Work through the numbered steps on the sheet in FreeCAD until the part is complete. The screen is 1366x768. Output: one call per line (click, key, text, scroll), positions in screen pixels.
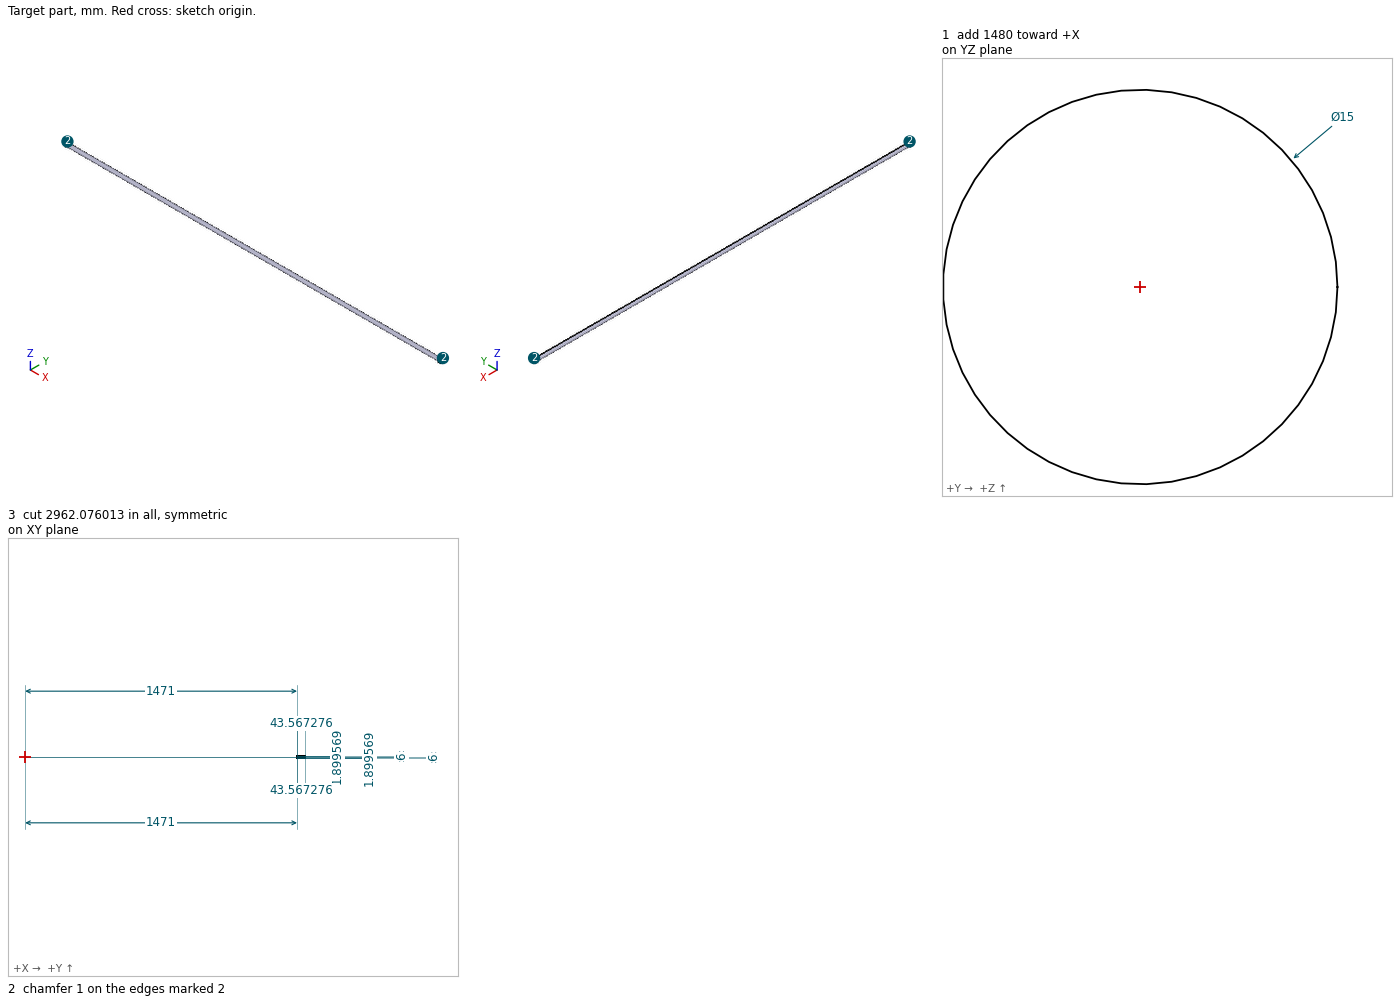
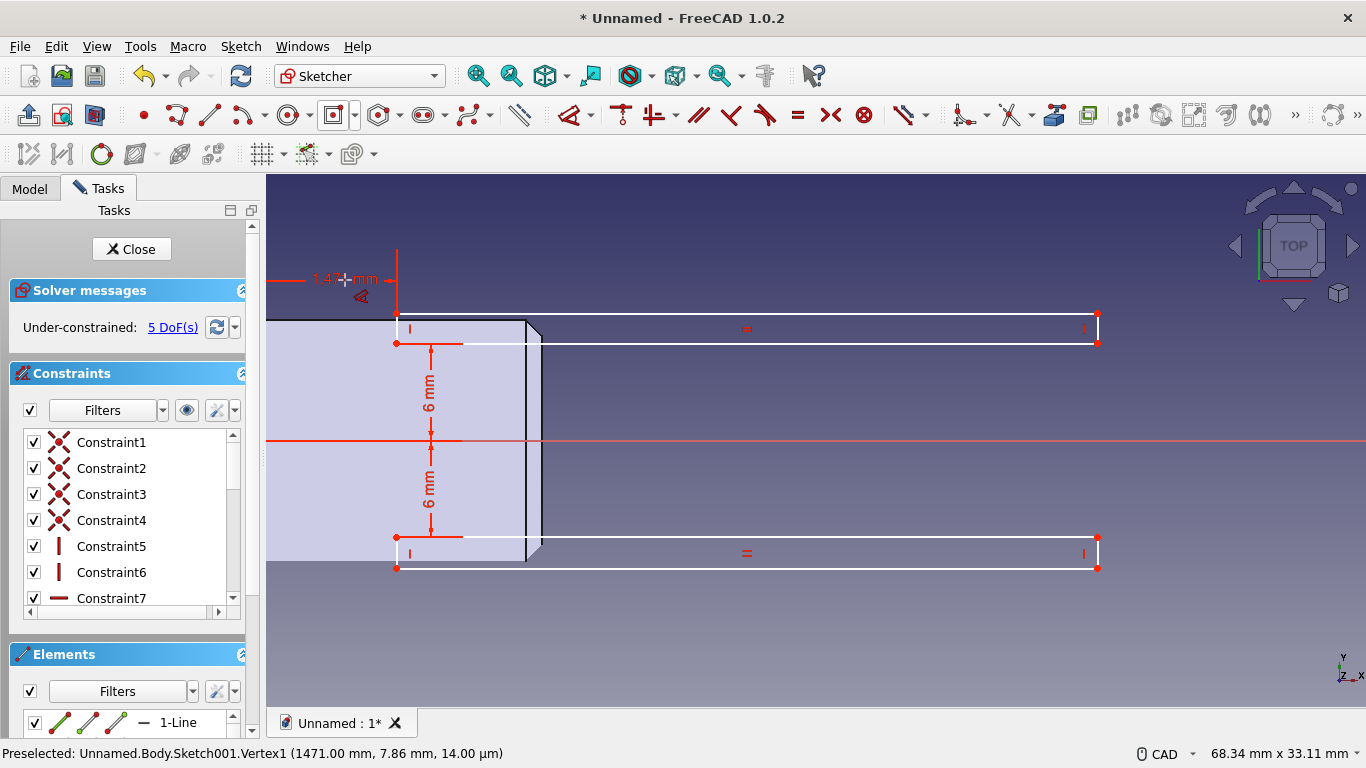
click(397, 537)
click(345, 571)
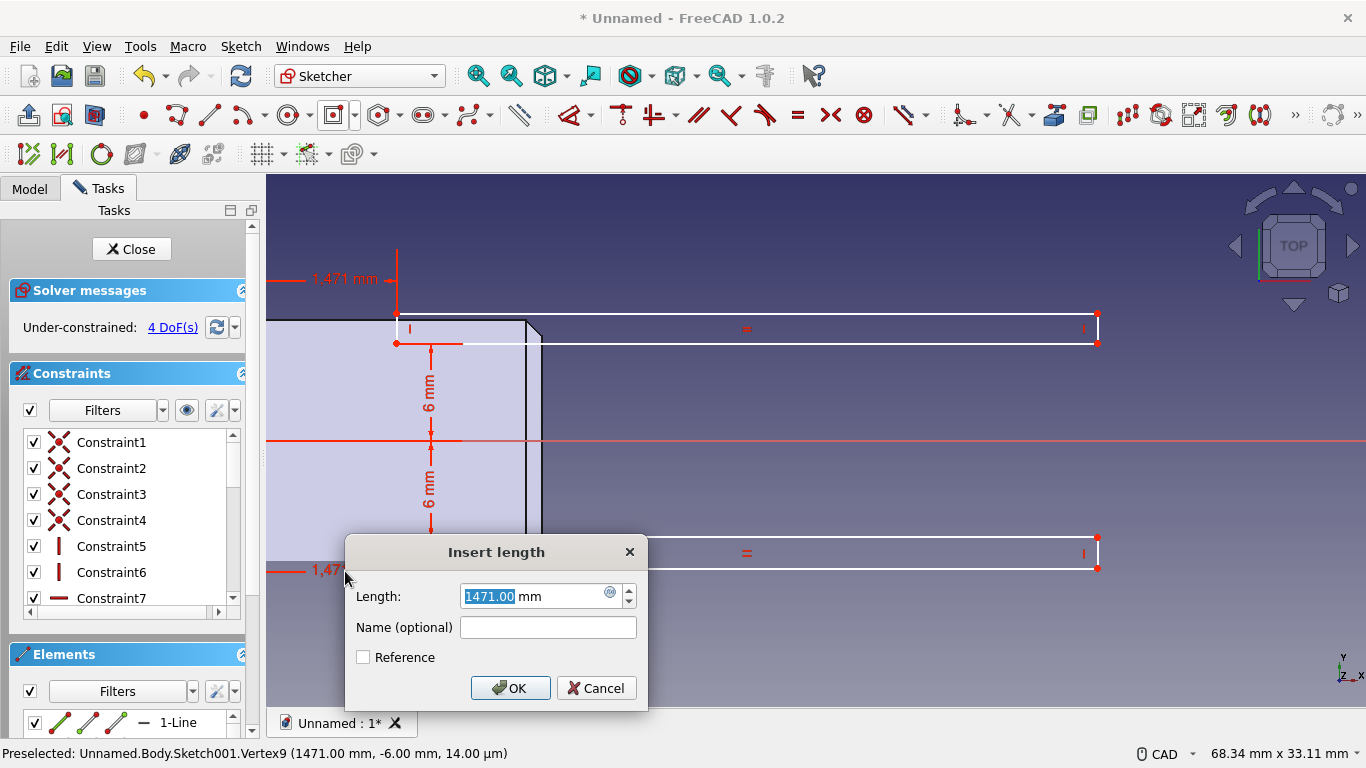
text(1471)
key(Return)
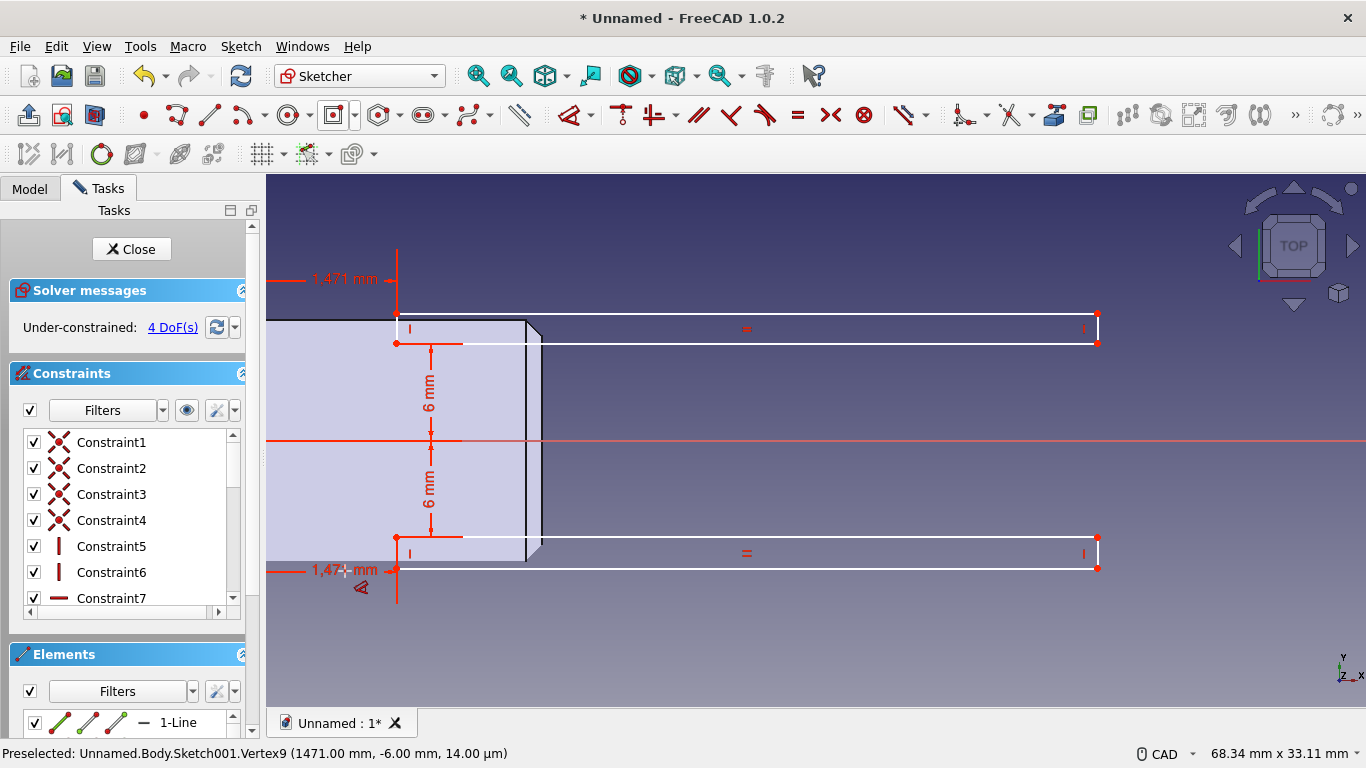
scroll(397, 326, up, 2)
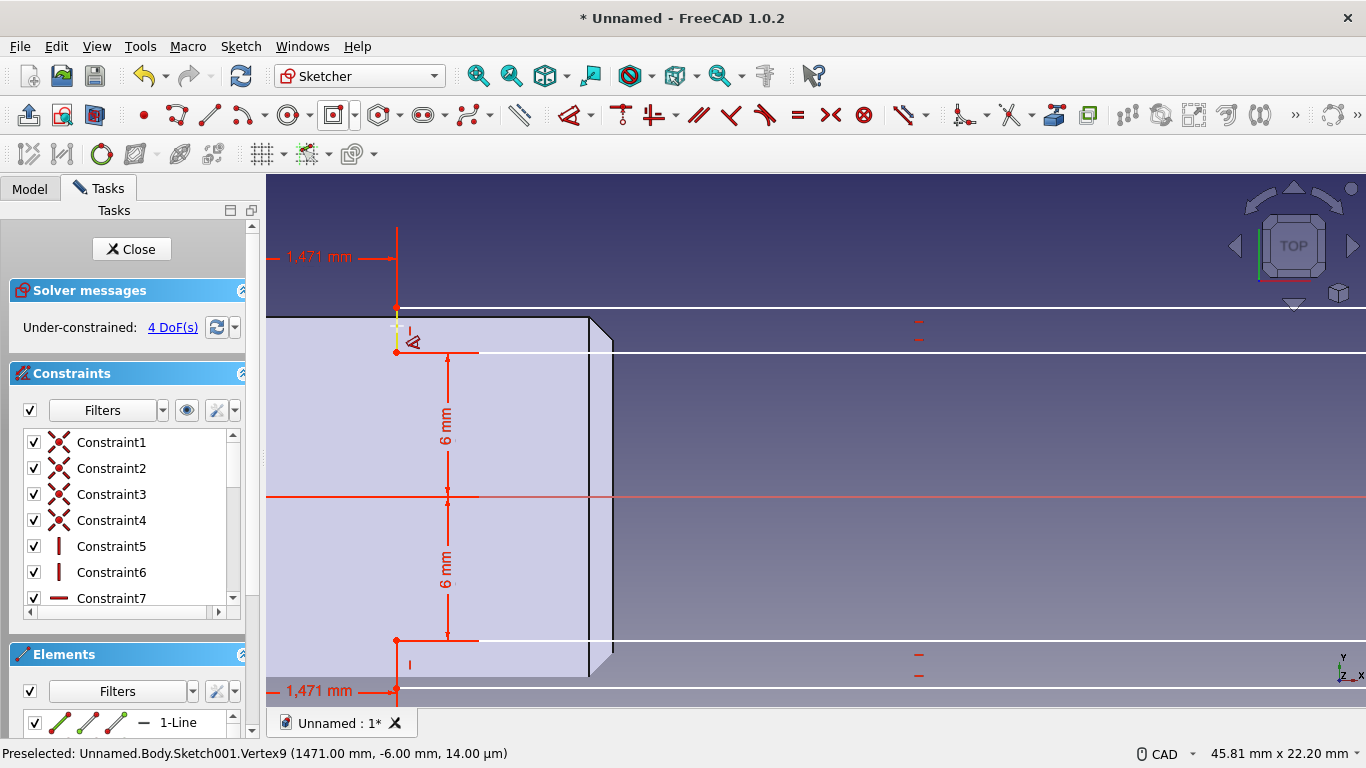
click(397, 326)
click(363, 330)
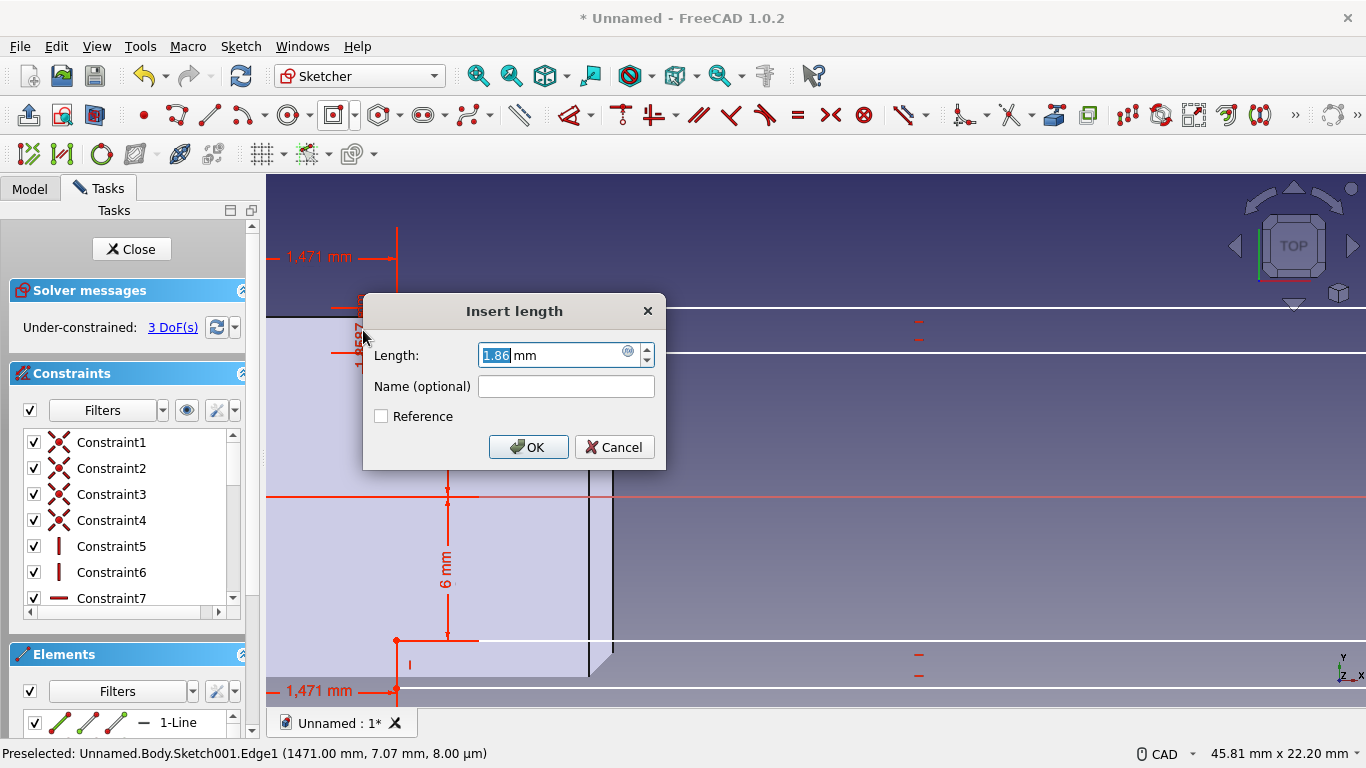
text(1.899569)
key(Return)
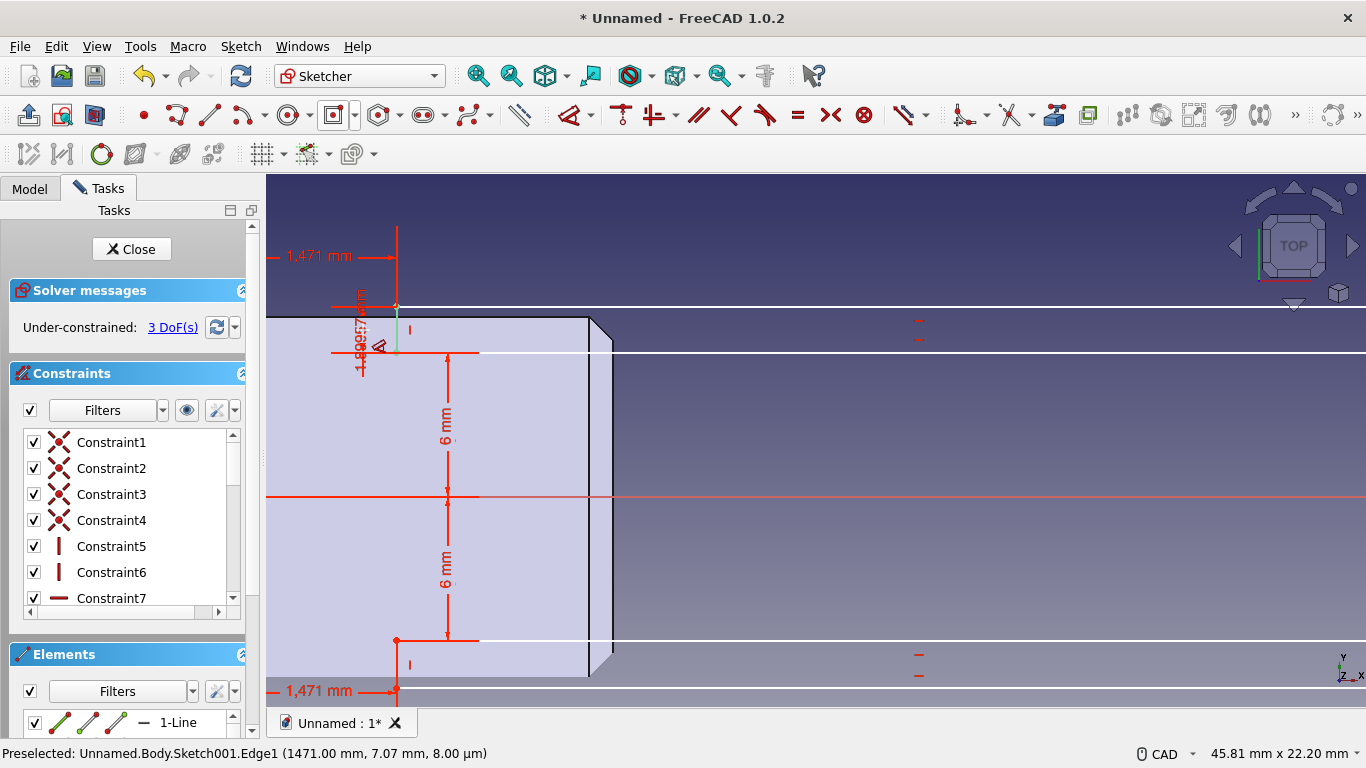
click(397, 655)
click(363, 660)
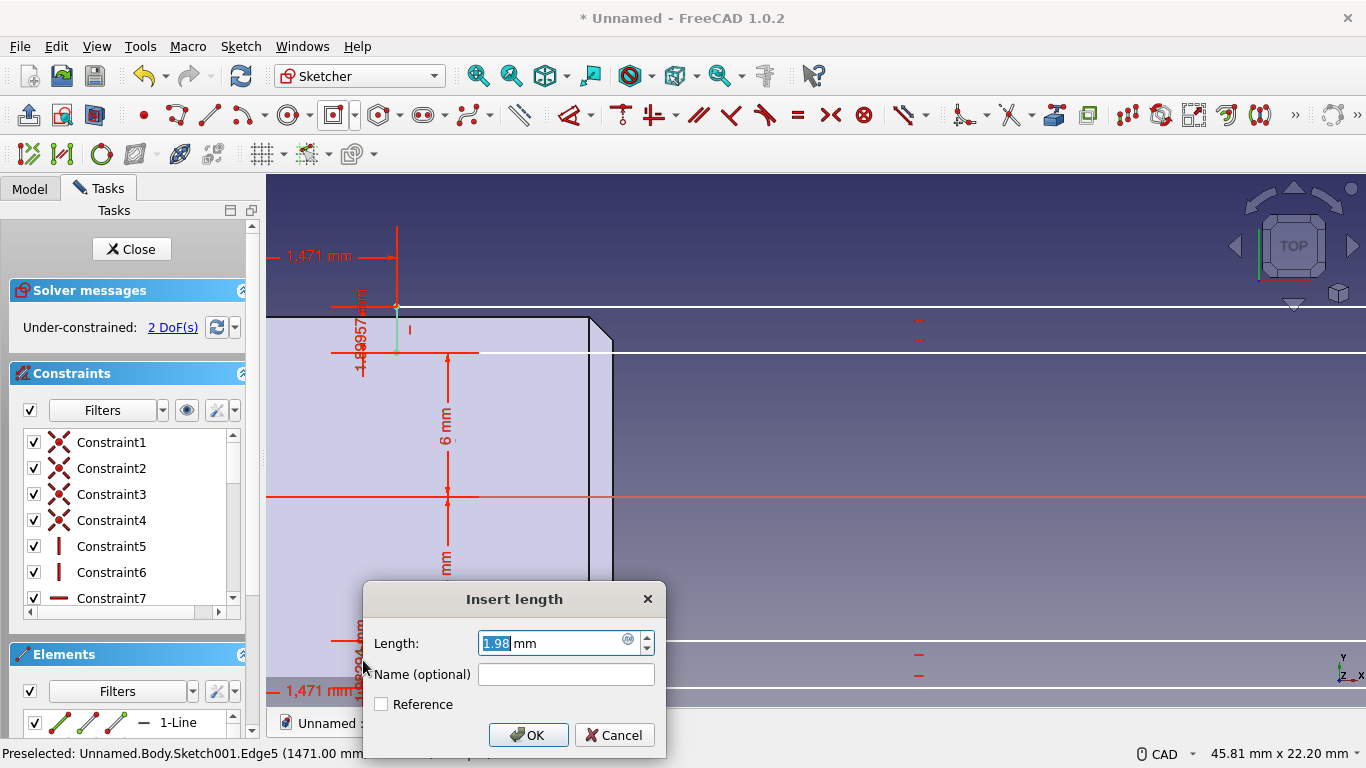
text(1.899569)
key(Return)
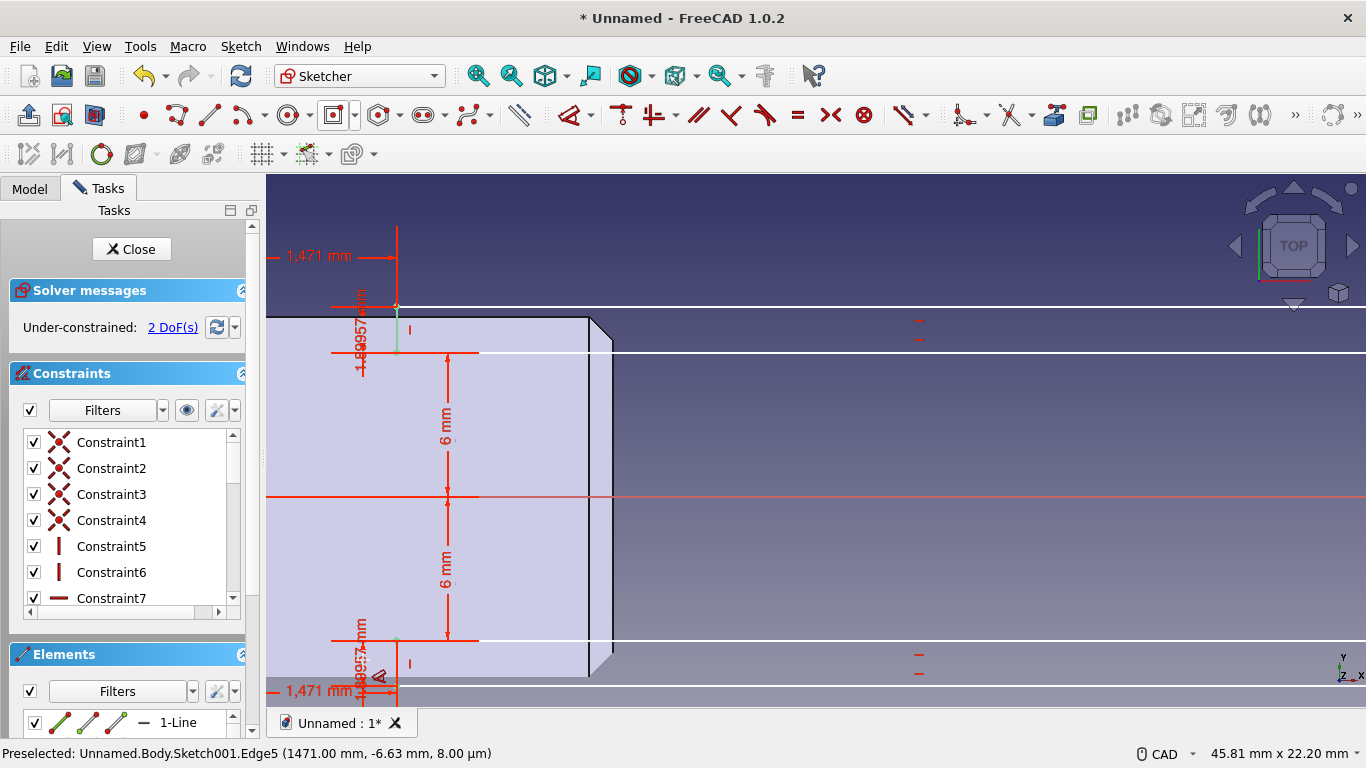
click(711, 353)
click(799, 387)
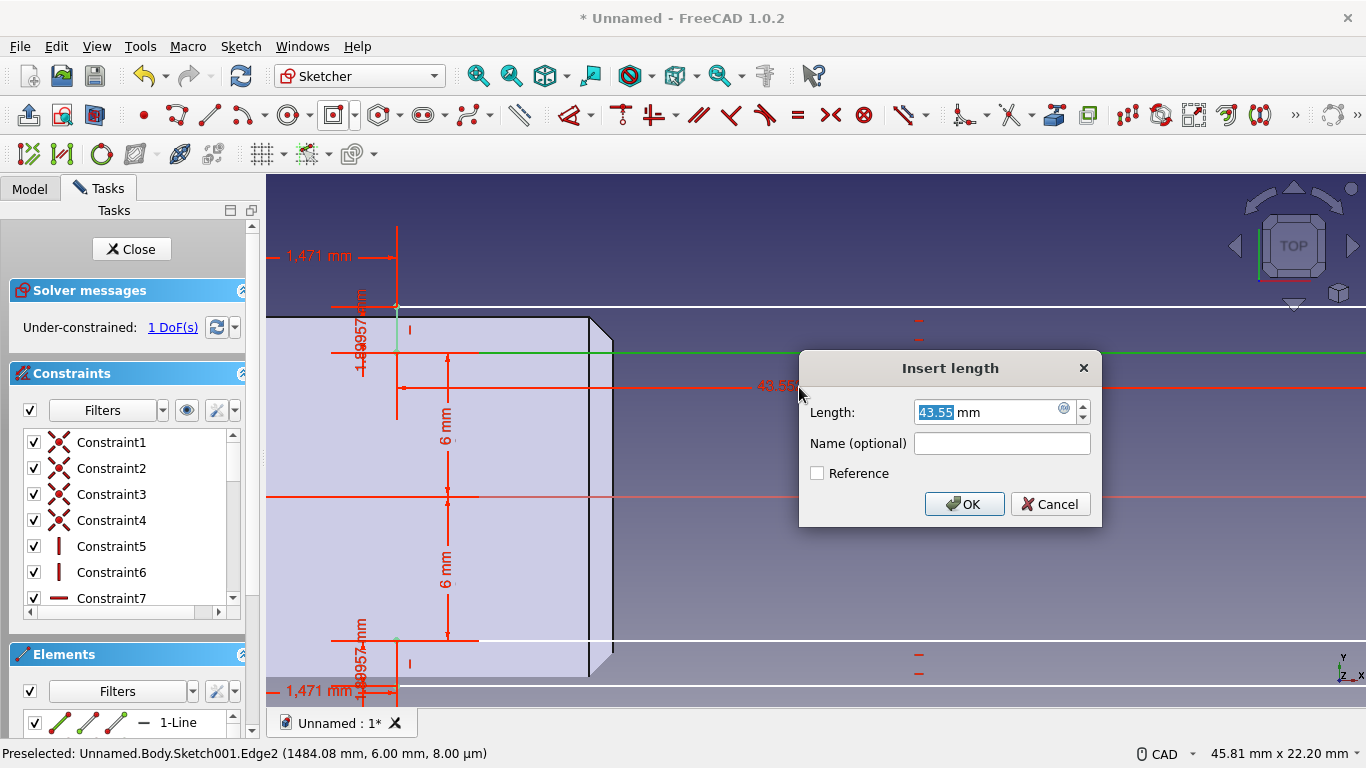
text(43.567276)
key(Return)